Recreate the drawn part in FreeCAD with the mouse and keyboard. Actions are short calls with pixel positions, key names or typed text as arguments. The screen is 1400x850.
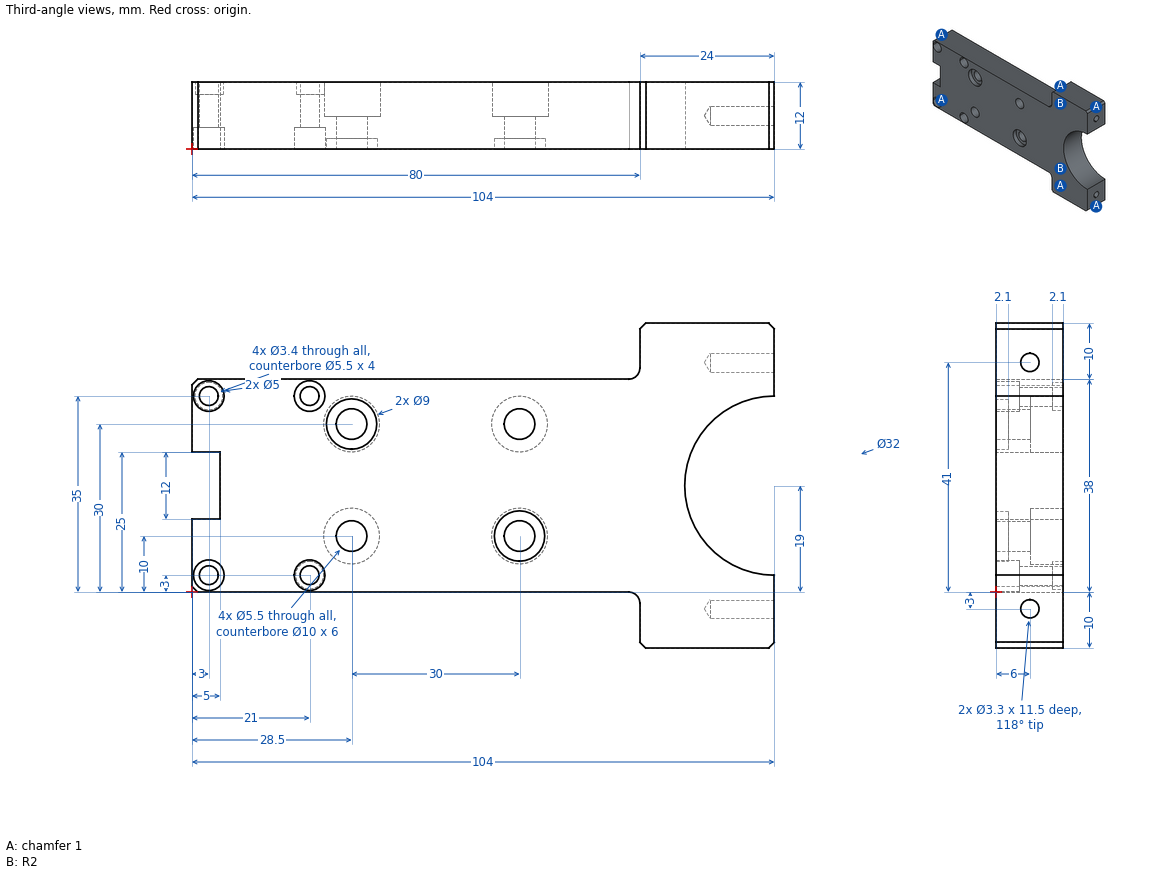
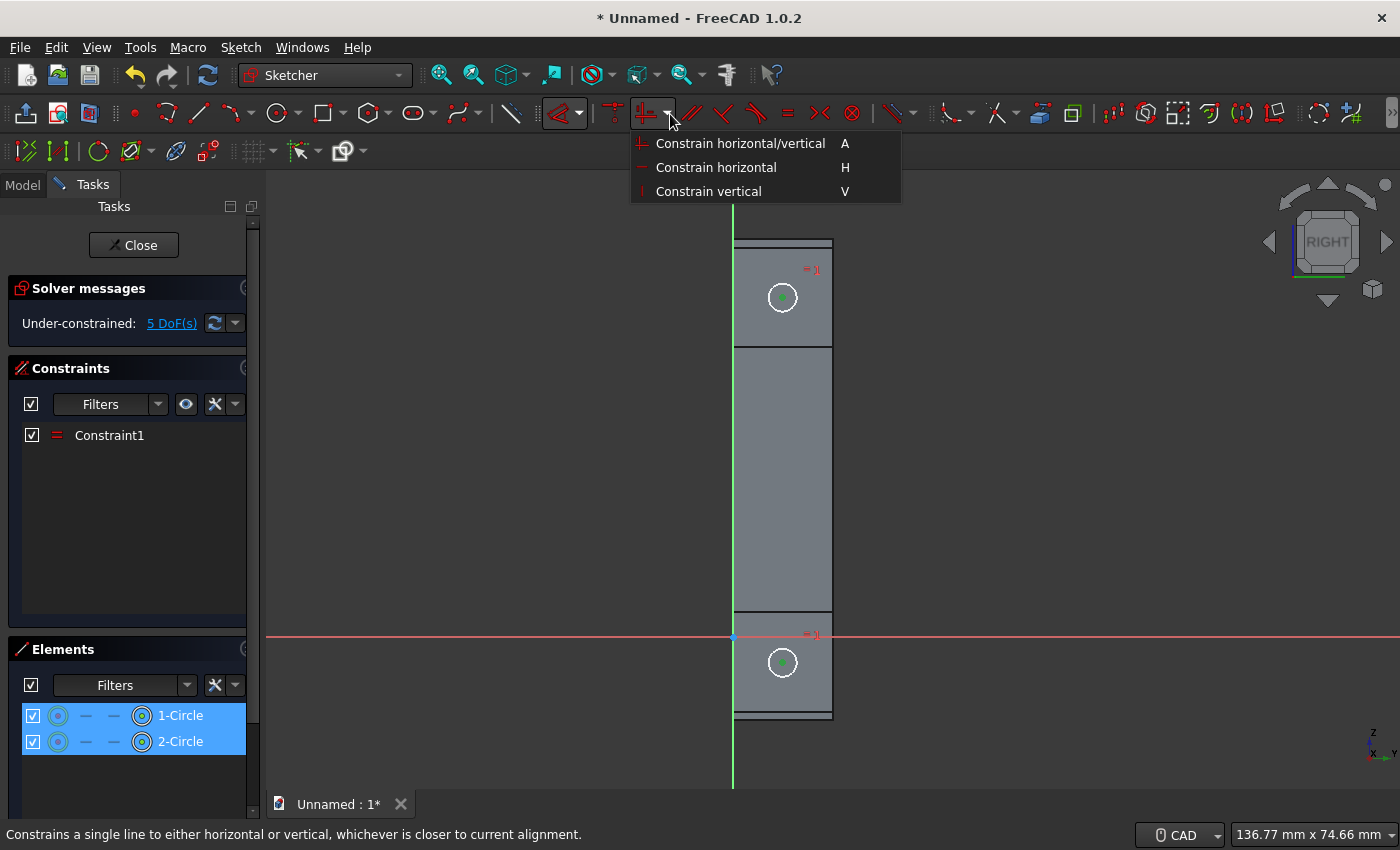
click(766, 191)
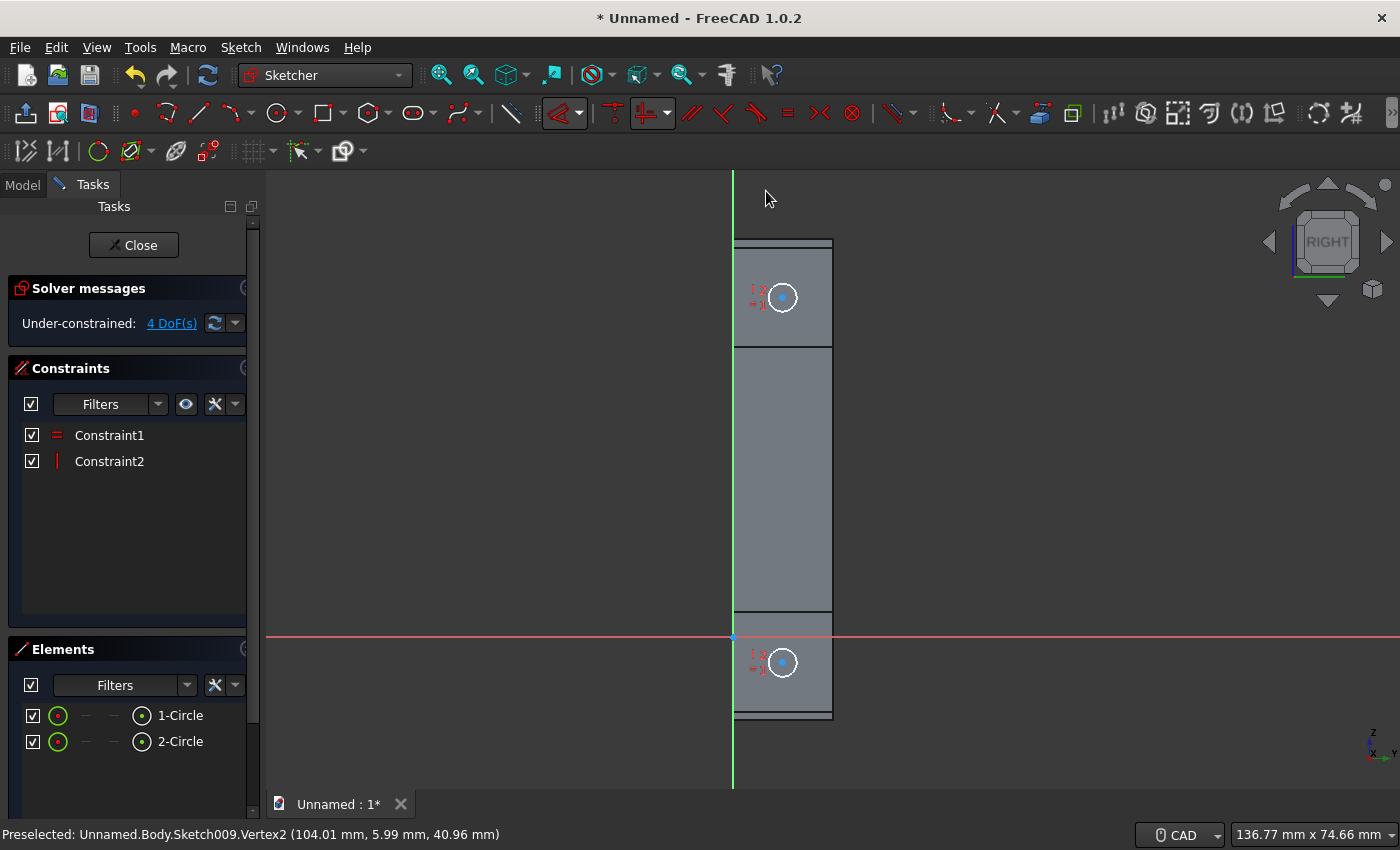
scroll(793, 653, up, 2)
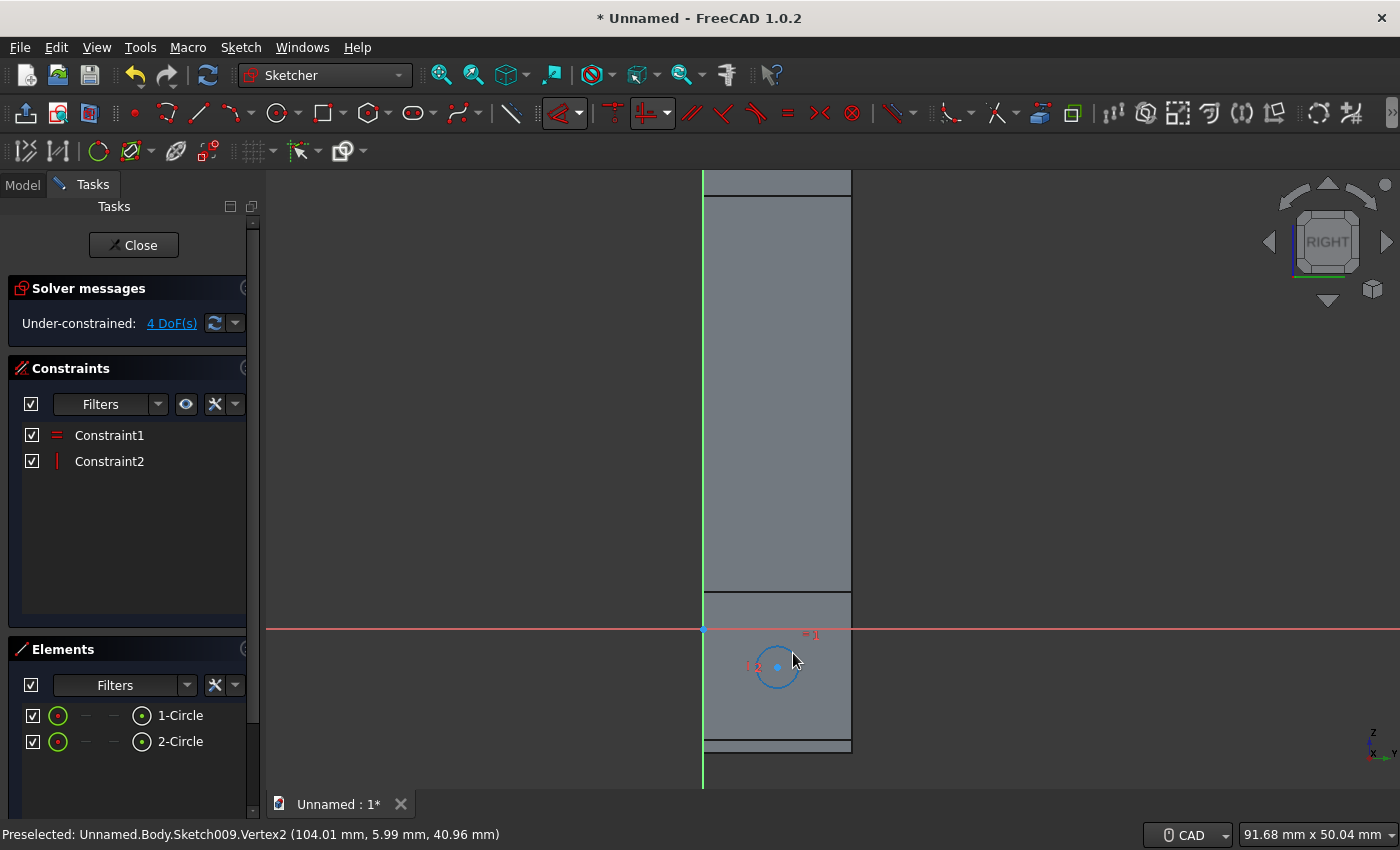
click(792, 652)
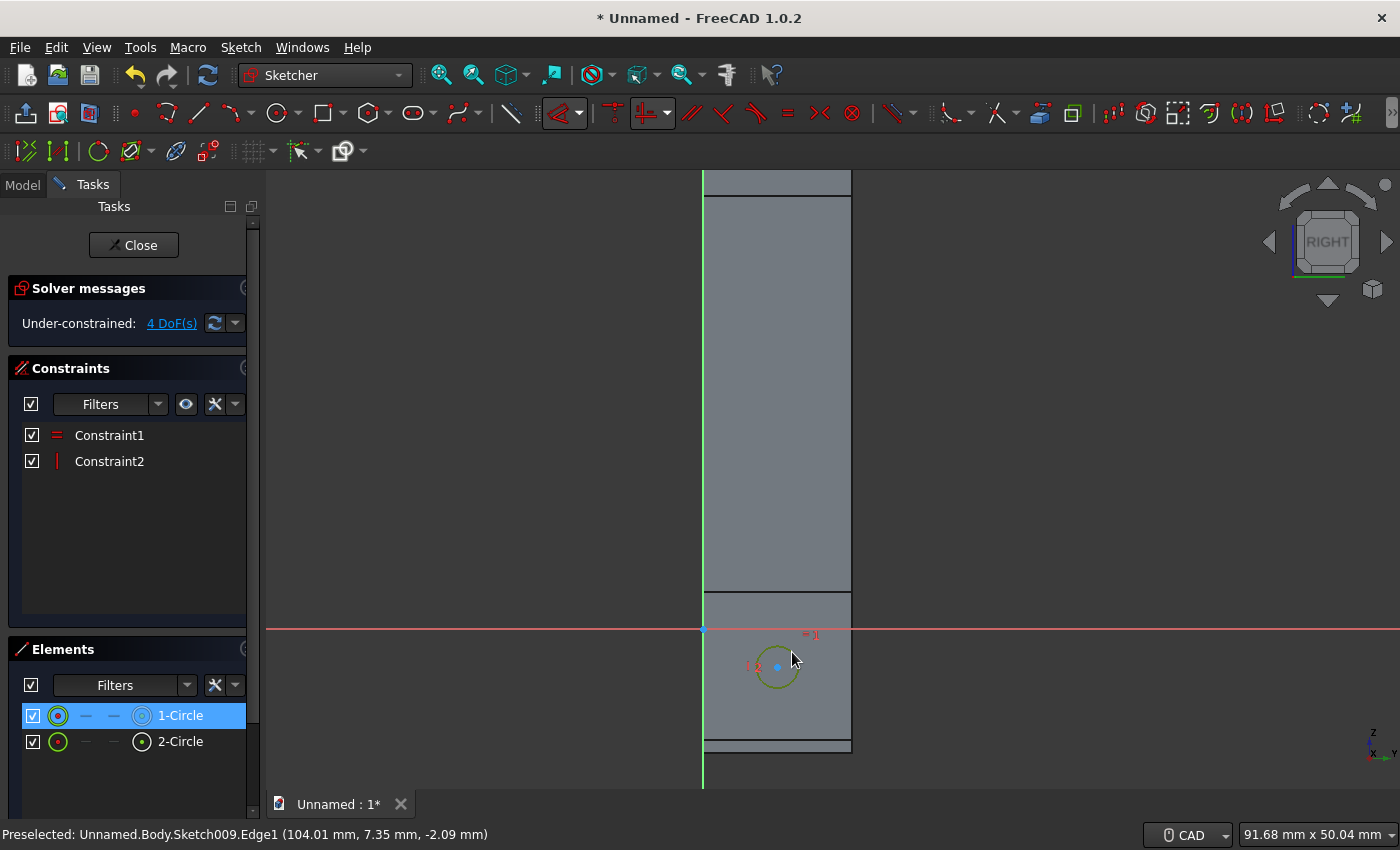
click(582, 114)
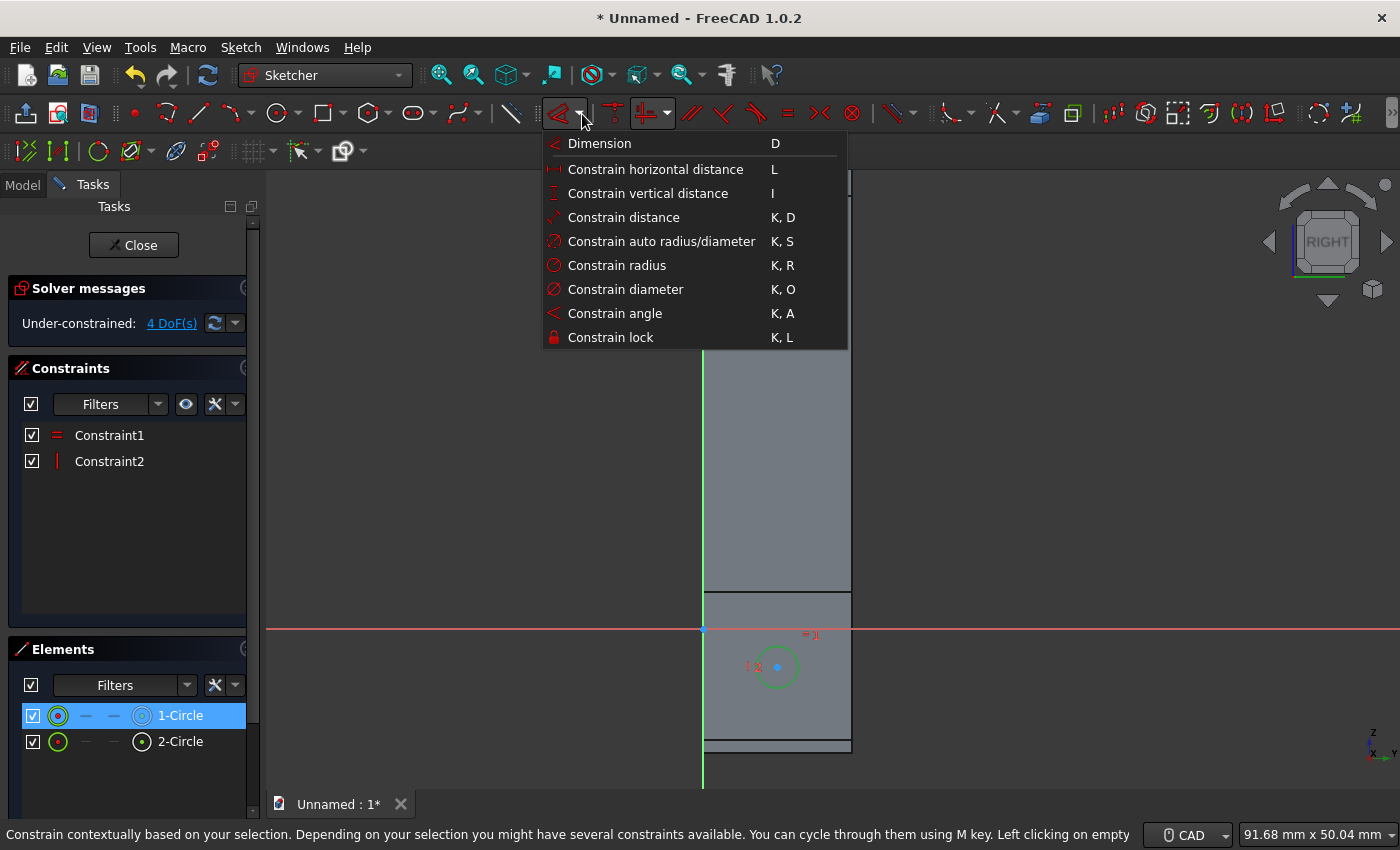
click(695, 289)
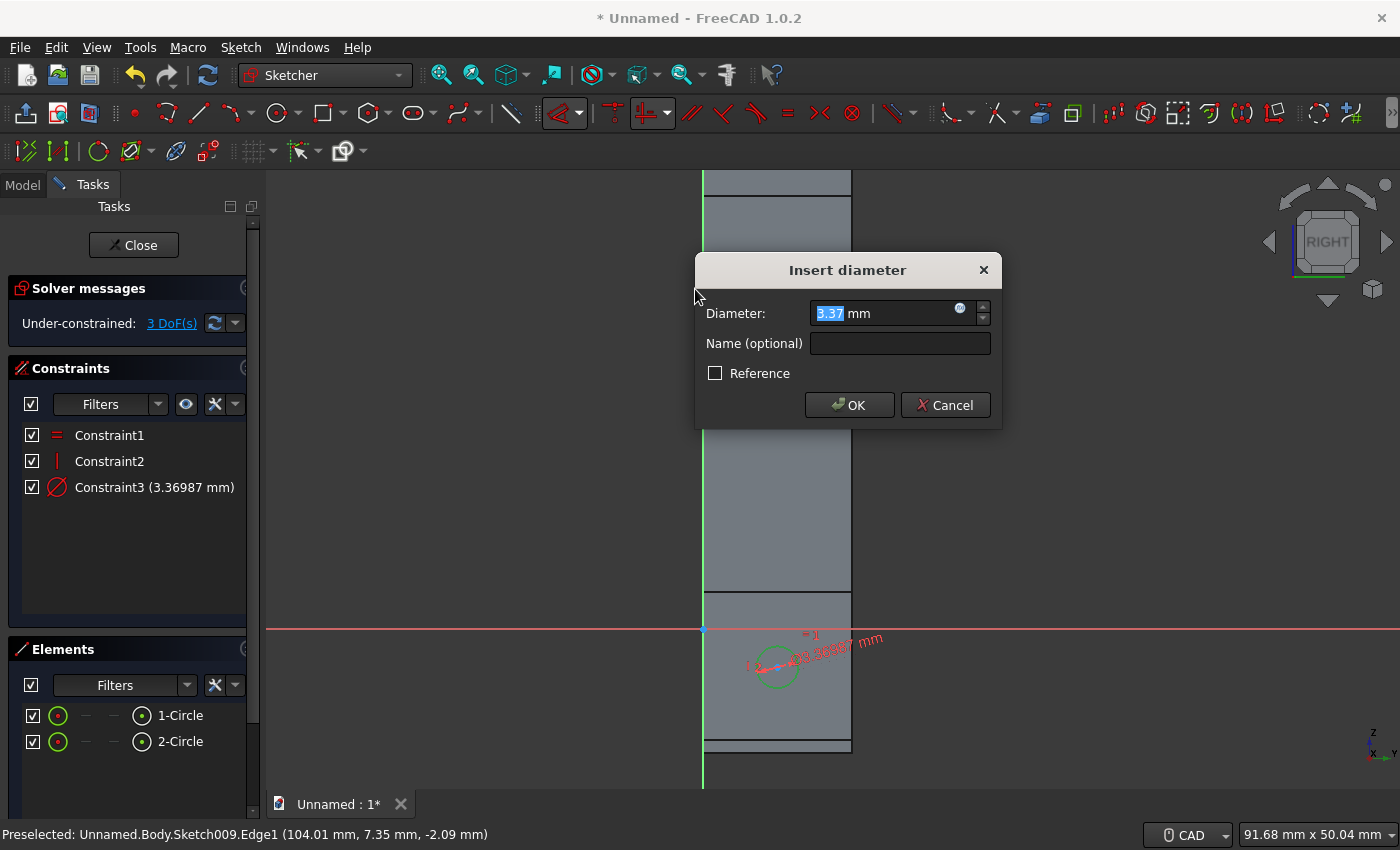
text(3.3)
key(Return)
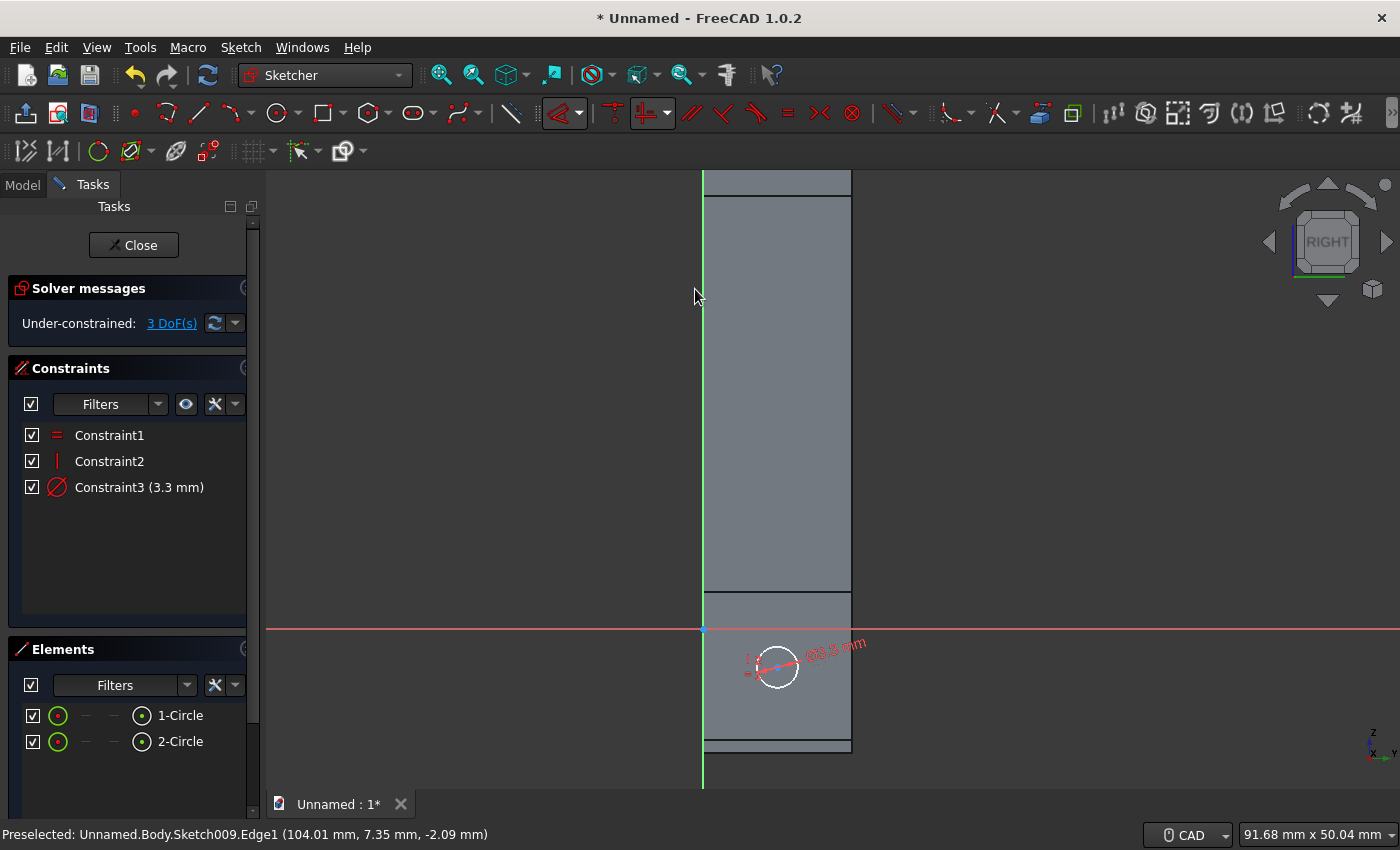
click(777, 667)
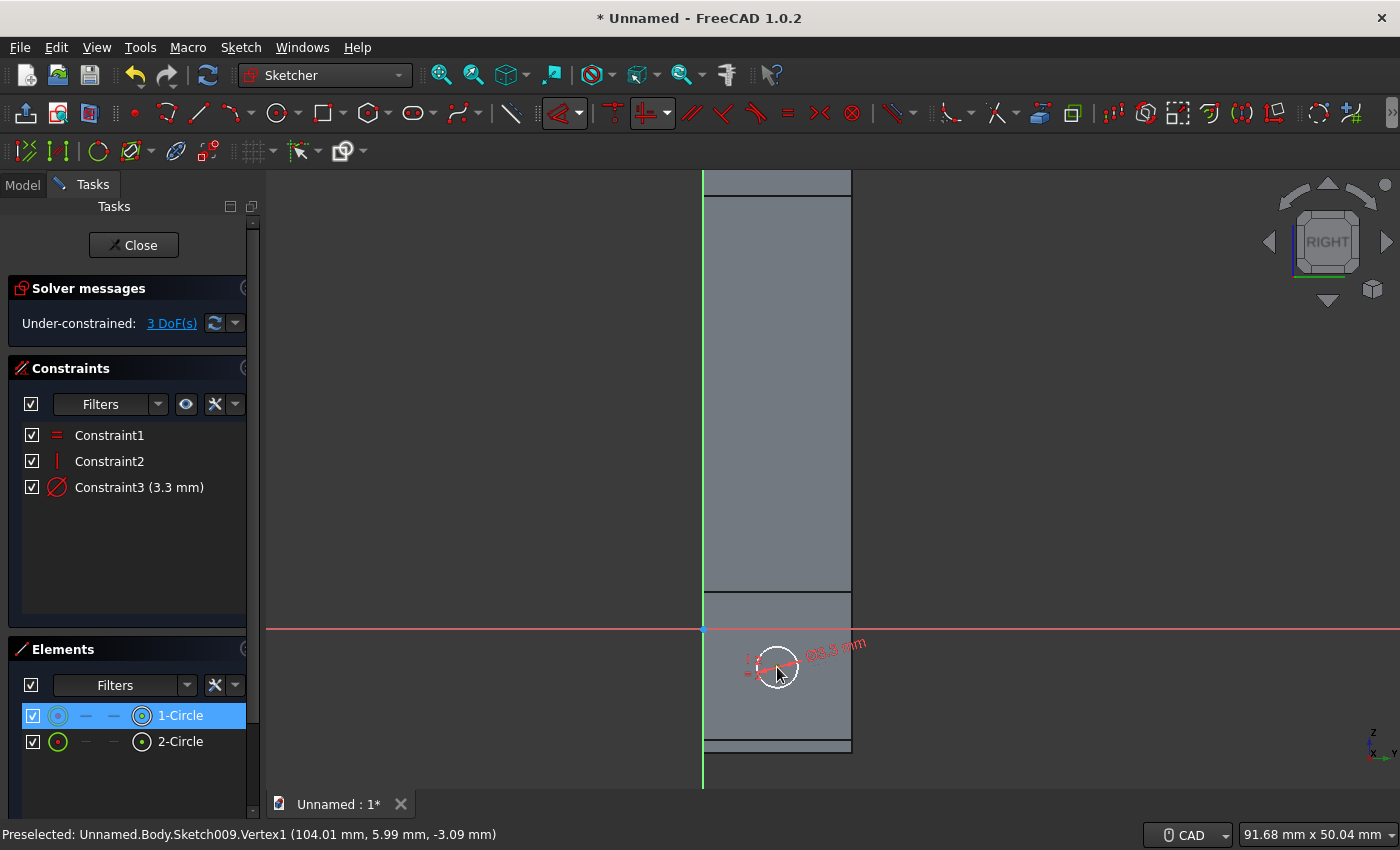
key(l)